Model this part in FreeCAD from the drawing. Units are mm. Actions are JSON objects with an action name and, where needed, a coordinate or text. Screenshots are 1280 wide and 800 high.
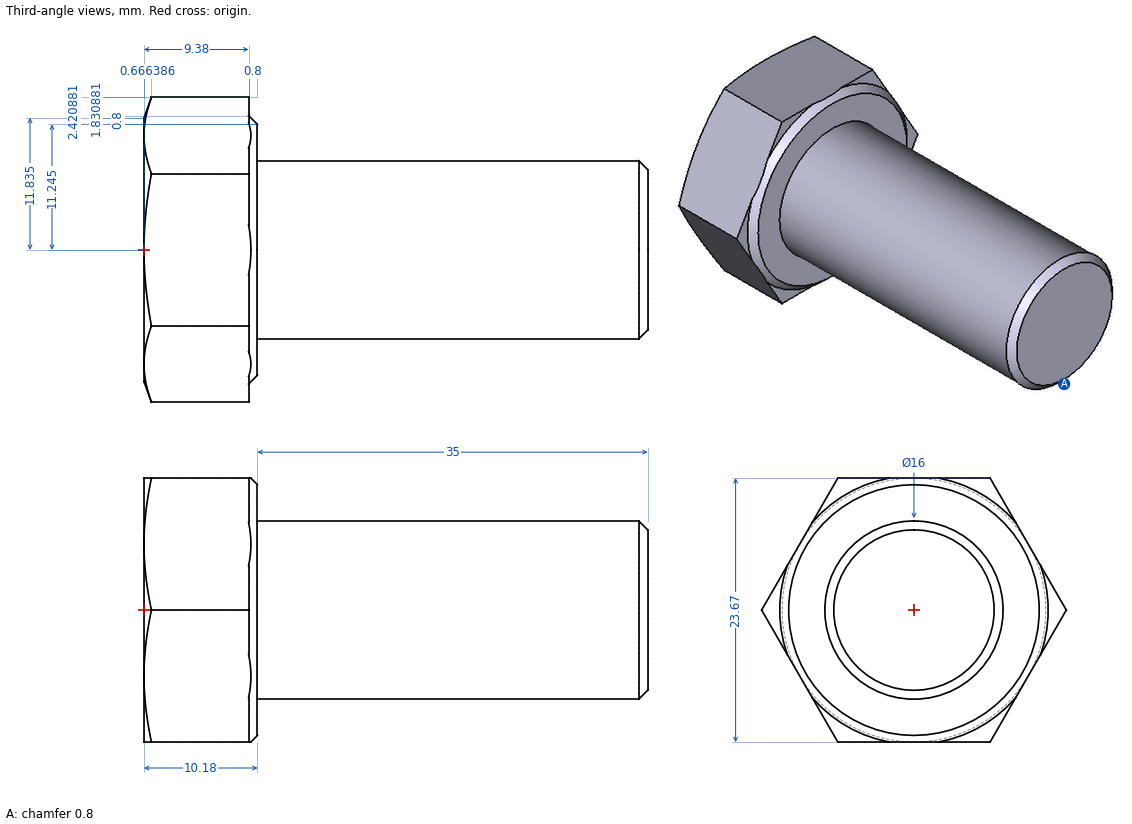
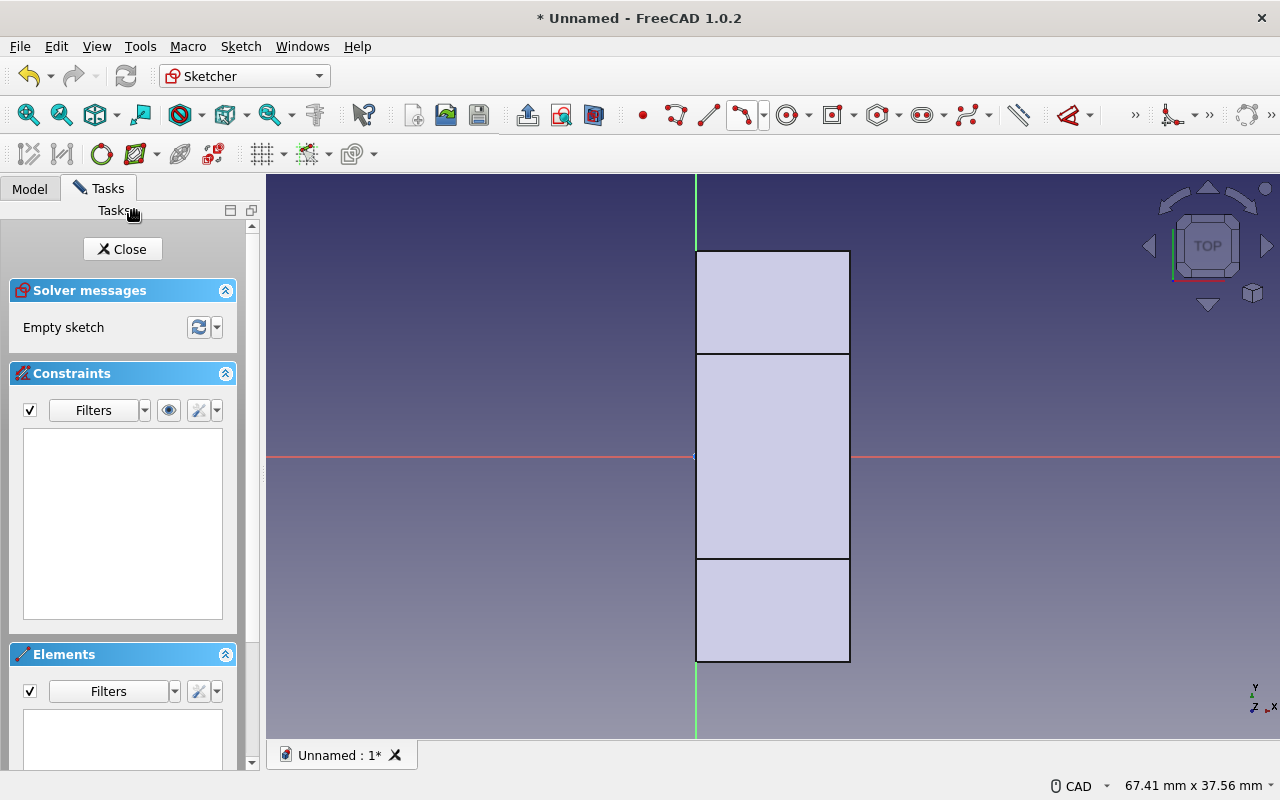
{"action": "left_click", "coordinate": [594, 116]}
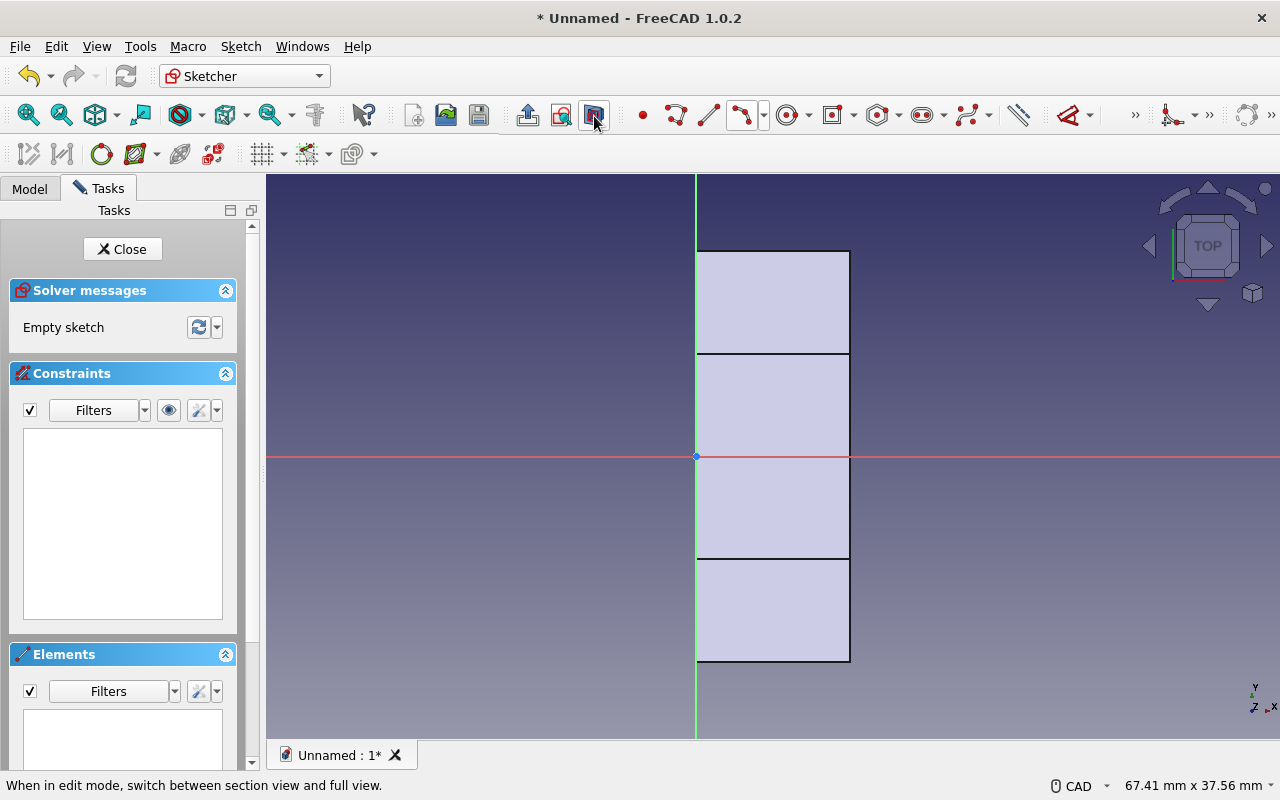
{"action": "scroll", "coordinate": [861, 246], "scroll_direction": "up", "scroll_amount": 11}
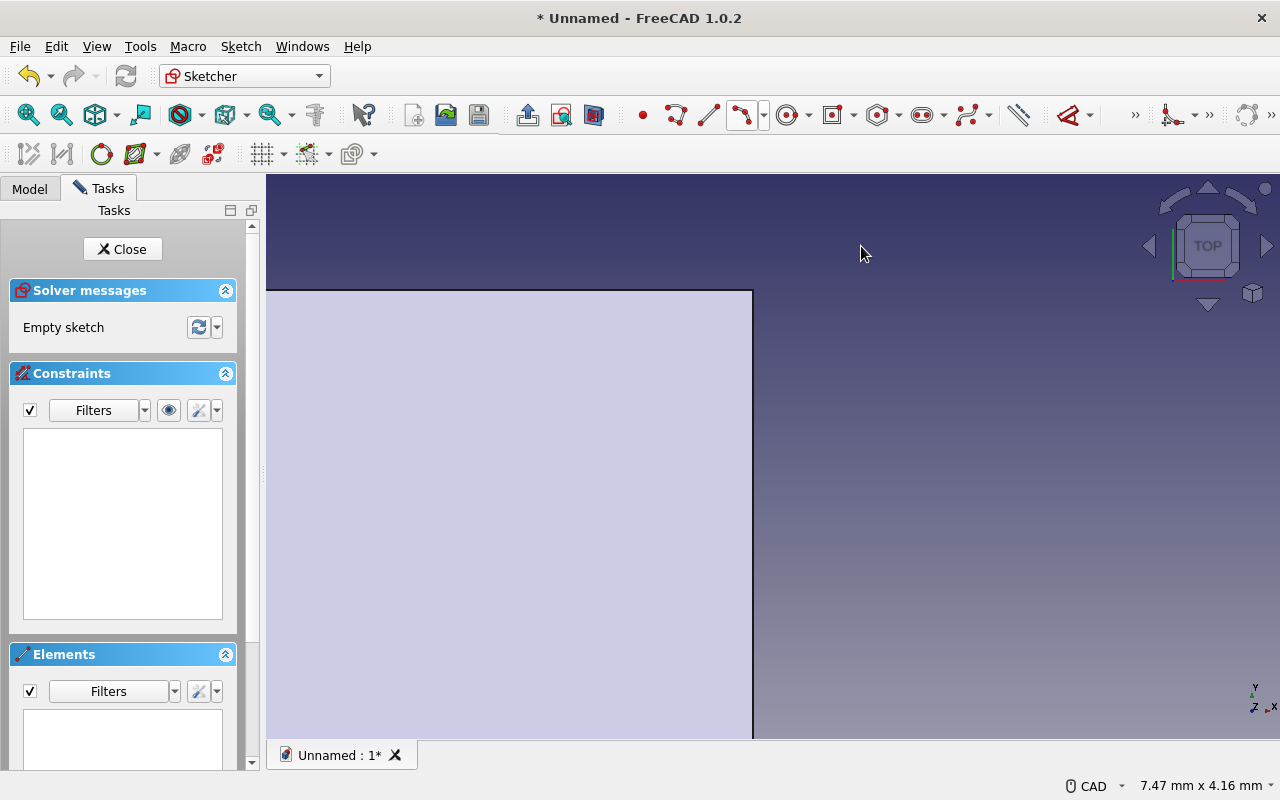
{"action": "left_click", "coordinate": [676, 116]}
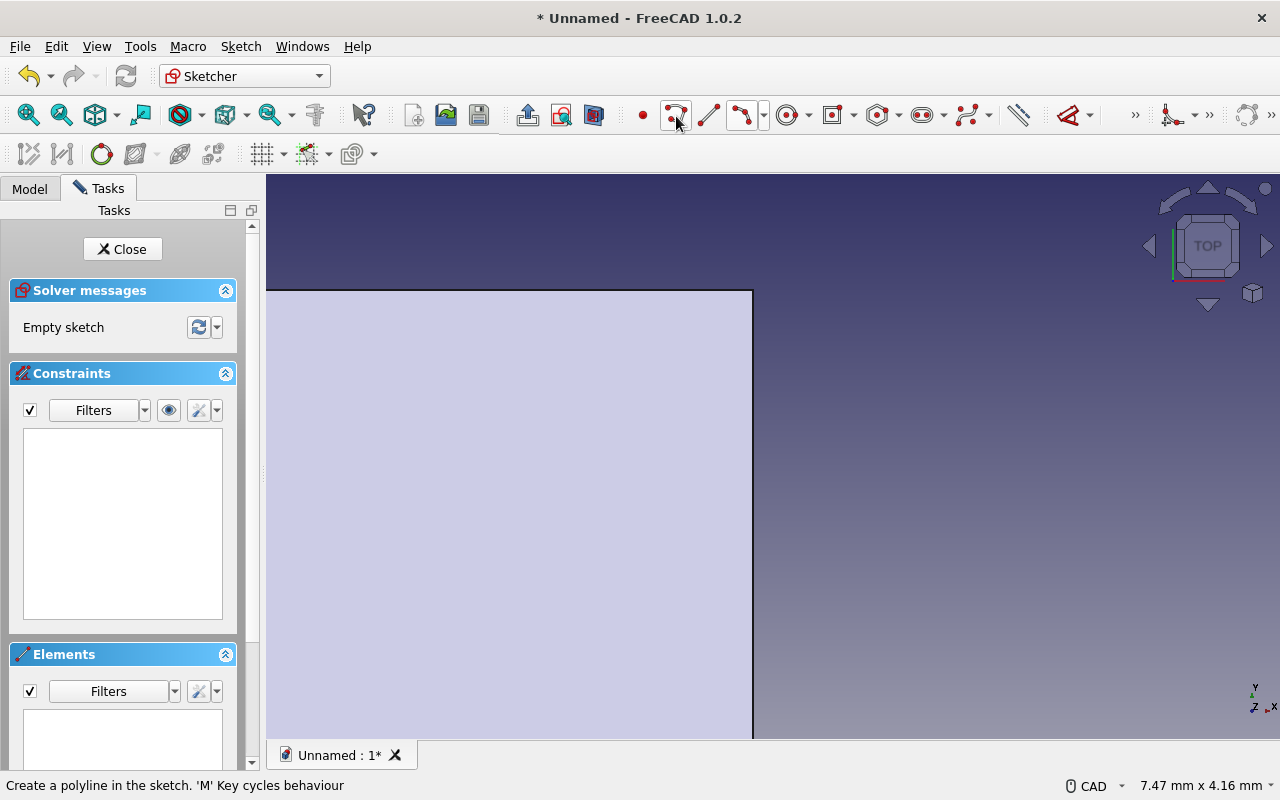
{"action": "left_click", "coordinate": [753, 618]}
{"action": "left_click", "coordinate": [753, 290]}
{"action": "left_click", "coordinate": [644, 290]}
{"action": "left_click", "coordinate": [644, 510]}
{"action": "left_click", "coordinate": [753, 619]}
{"action": "key", "text": "Escape"}
{"action": "key", "text": "Escape"}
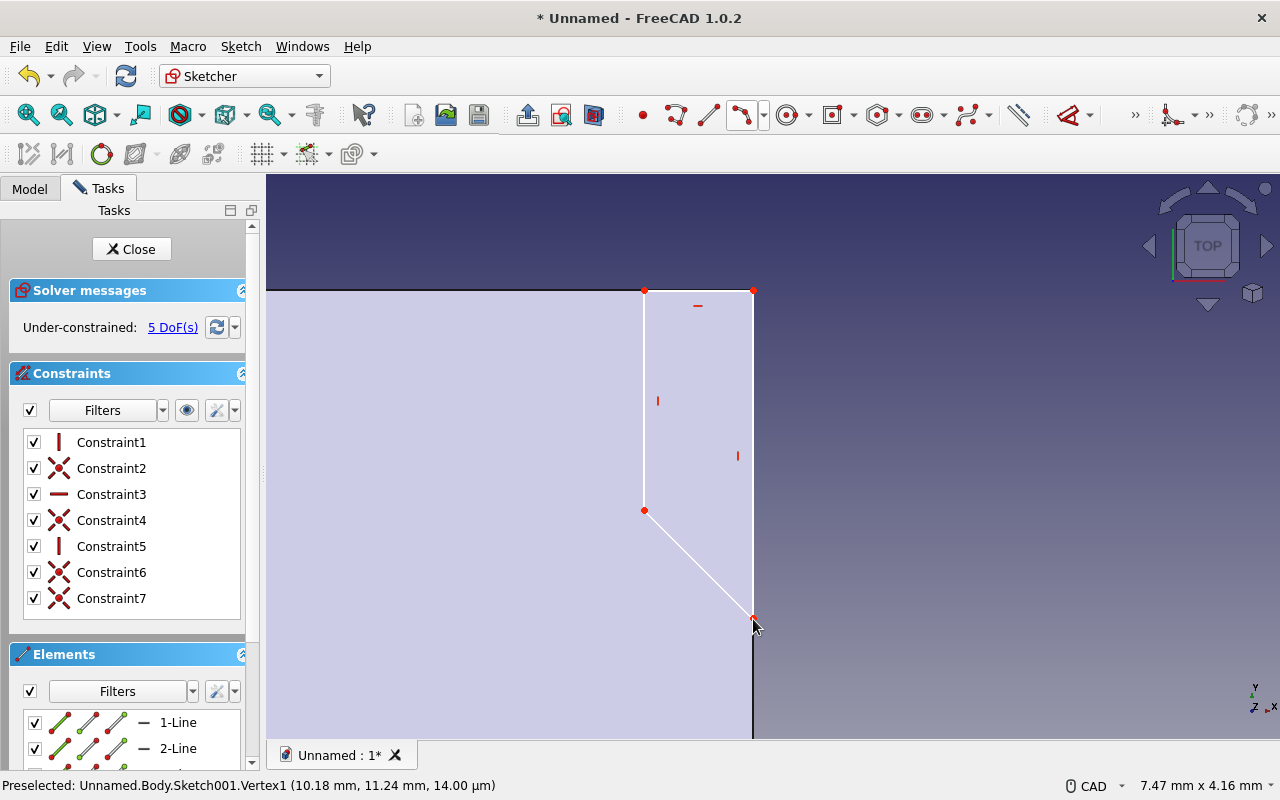
{"action": "key", "text": "d"}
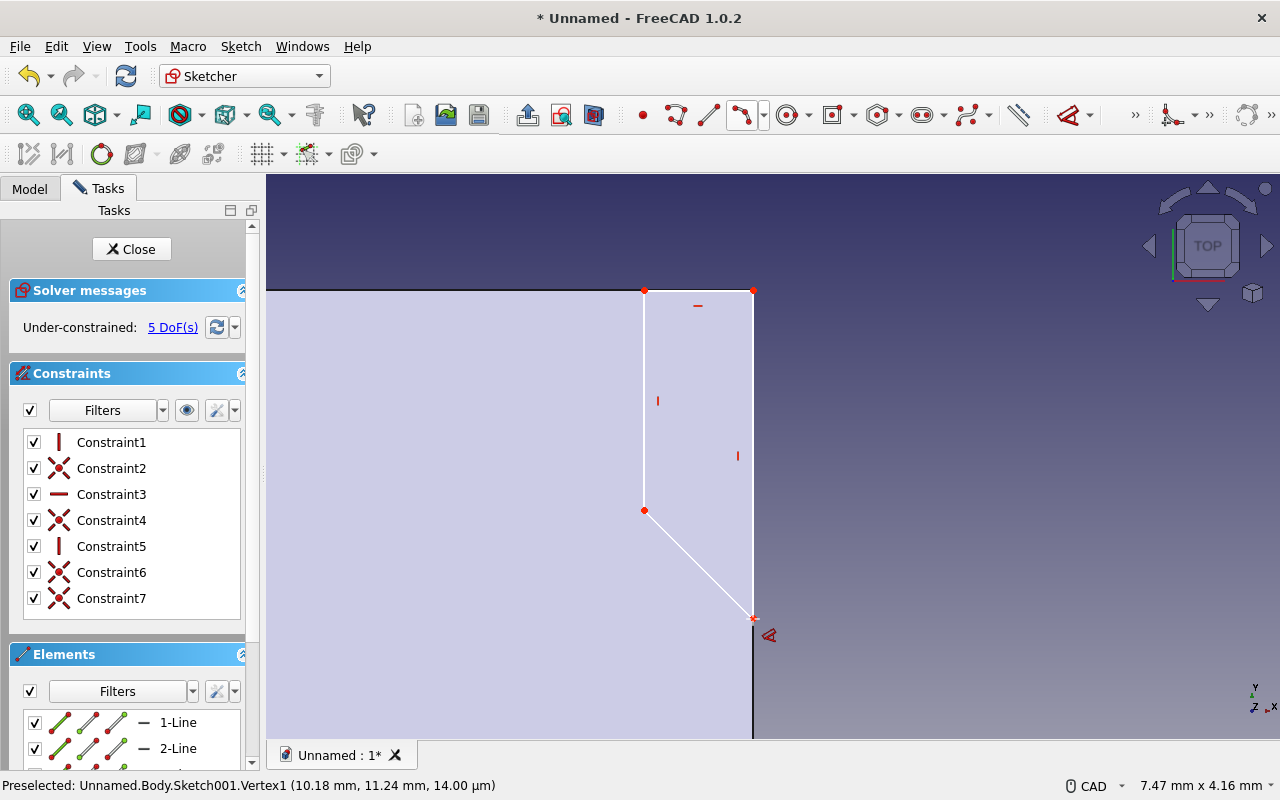
{"action": "left_click", "coordinate": [720, 291]}
{"action": "left_click", "coordinate": [699, 257]}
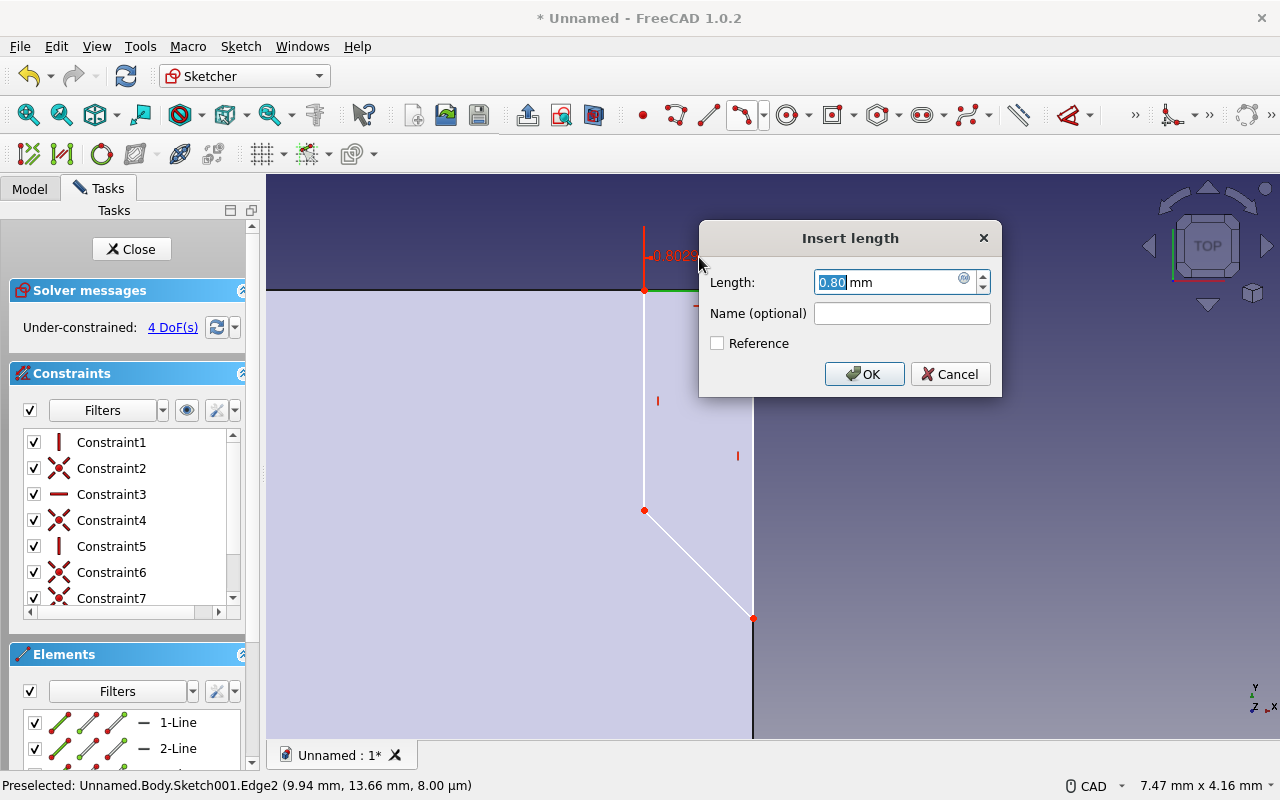
{"action": "type", "text": "0.8"}
{"action": "key", "text": "Return"}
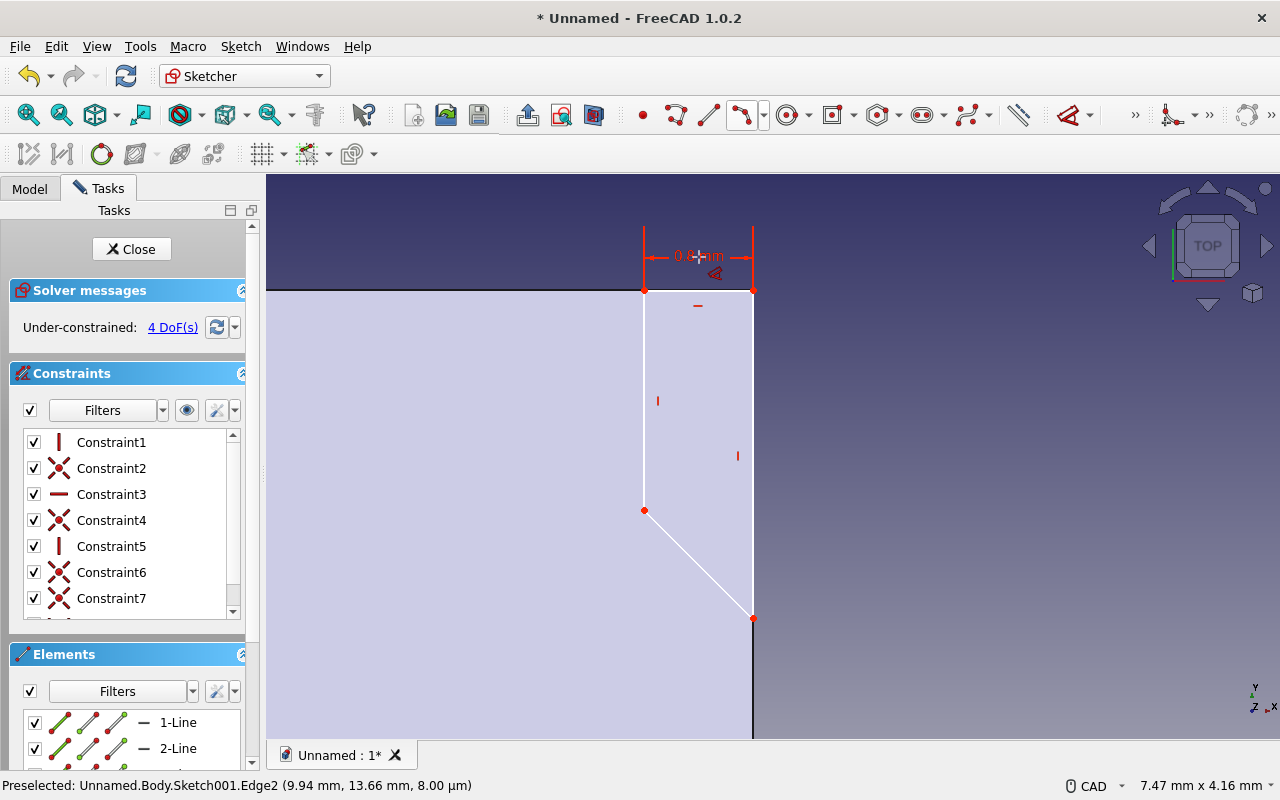
{"action": "left_click", "coordinate": [677, 543]}
{"action": "left_click", "coordinate": [610, 565]}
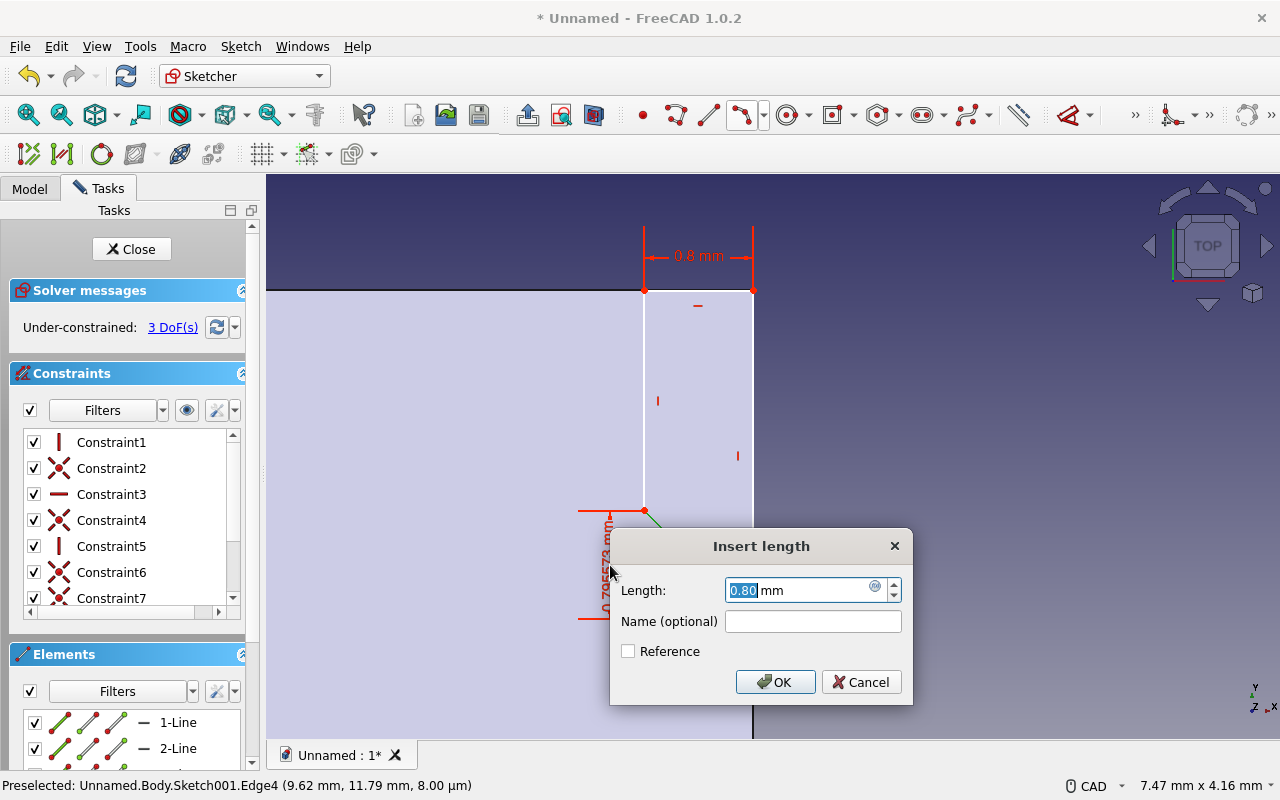
{"action": "type", "text": "0.8"}
{"action": "key", "text": "Return"}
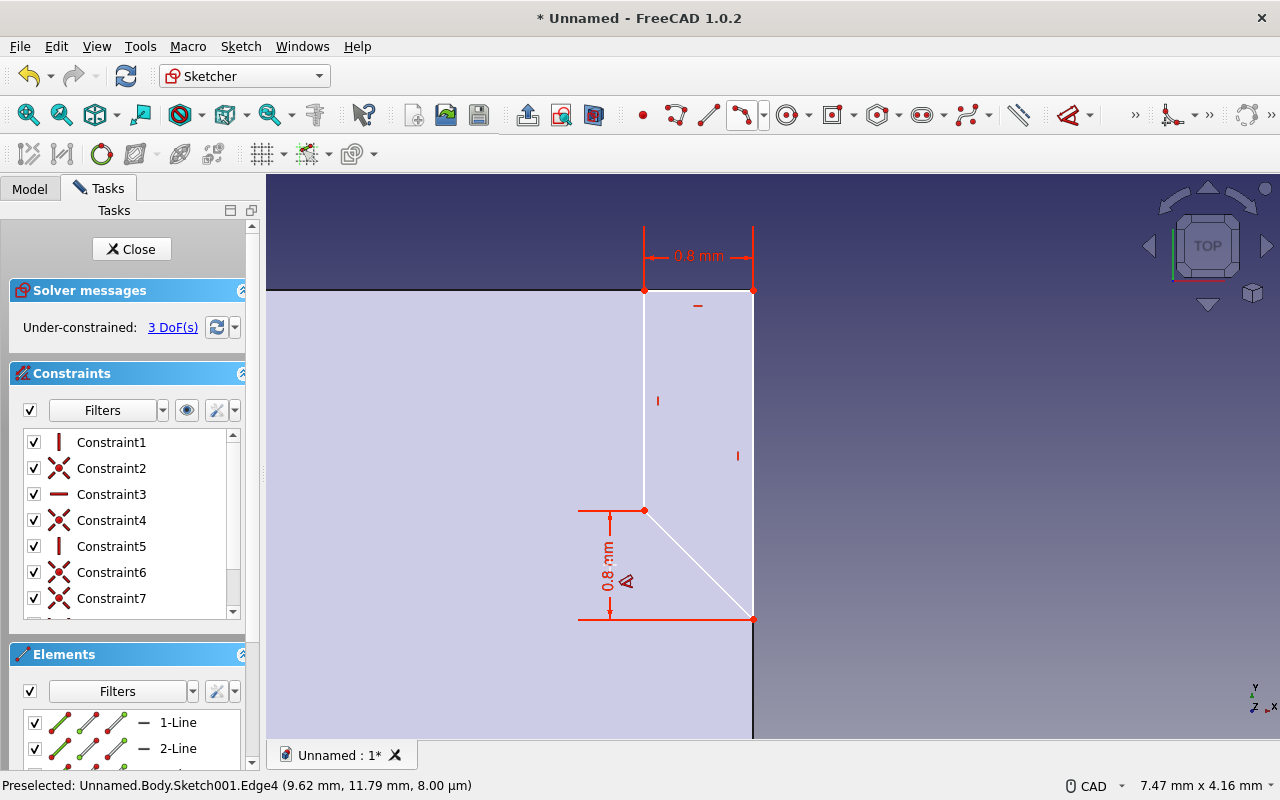
{"action": "left_click", "coordinate": [644, 291]}
{"action": "left_click", "coordinate": [469, 257]}